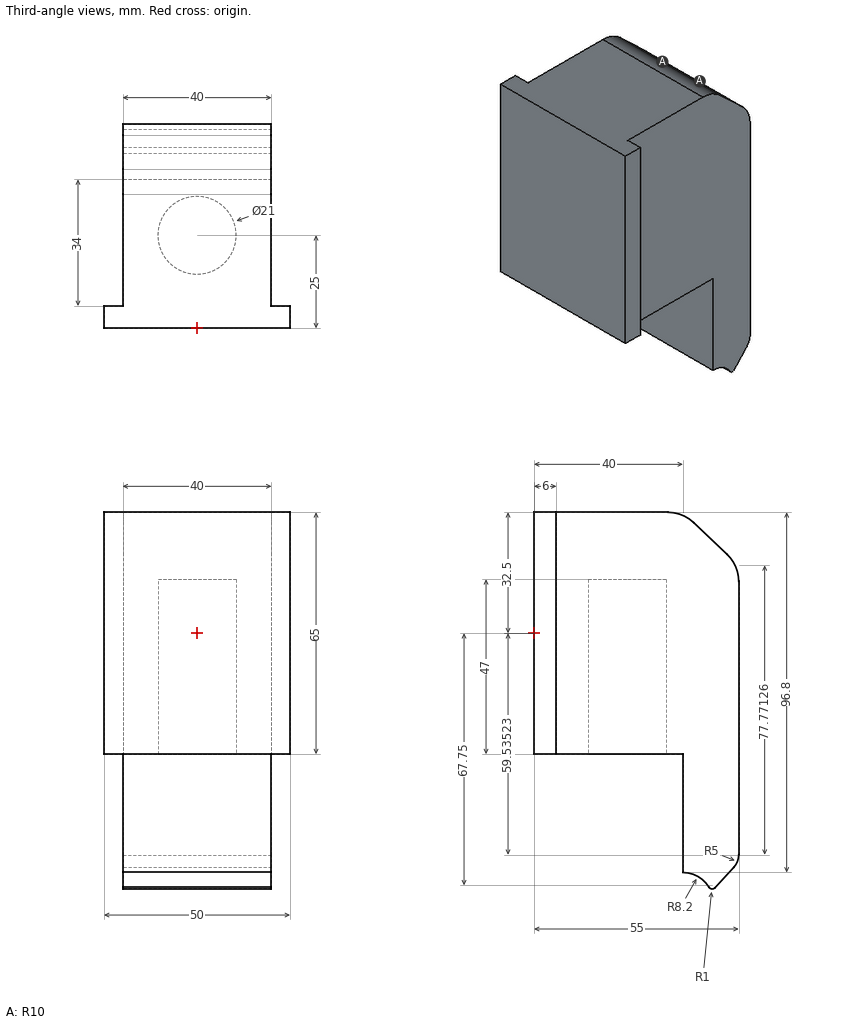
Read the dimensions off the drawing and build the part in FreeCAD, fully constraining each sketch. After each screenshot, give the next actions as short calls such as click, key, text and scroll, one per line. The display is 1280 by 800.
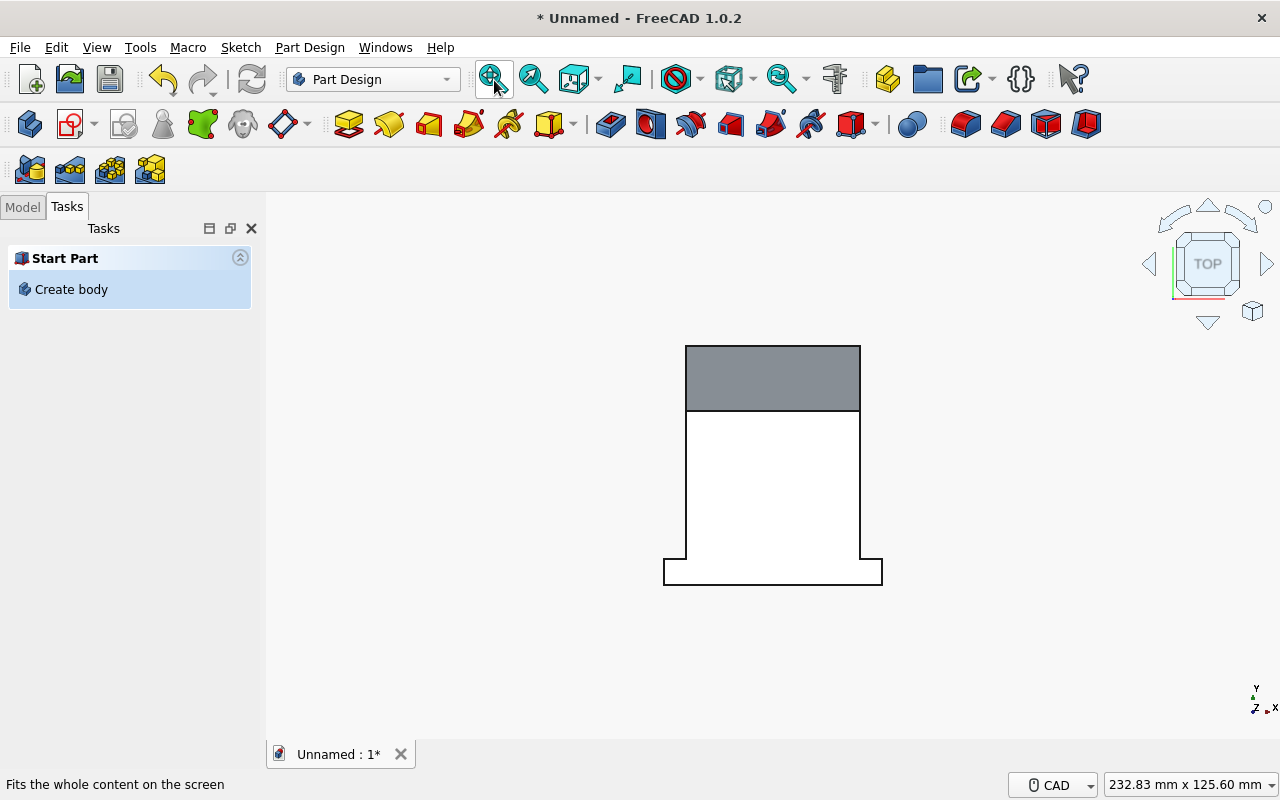
click(773, 410)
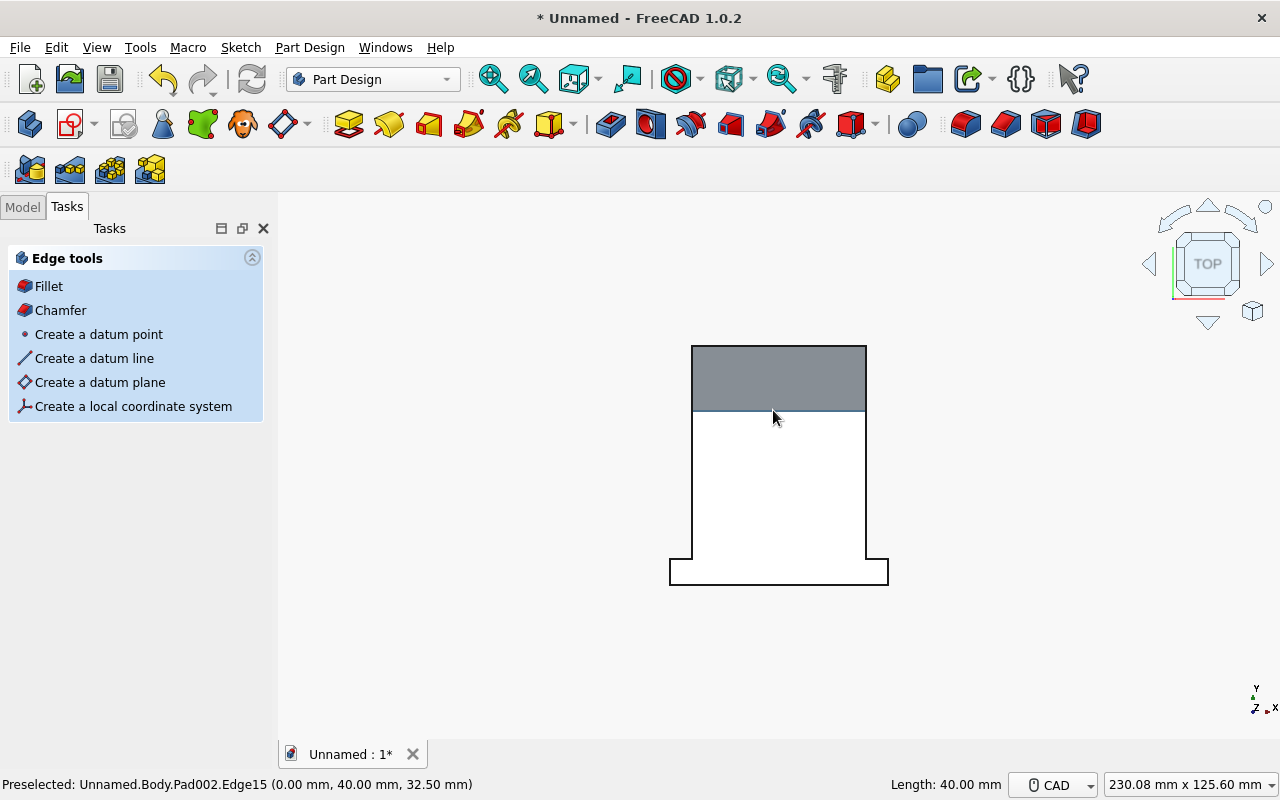
key(1)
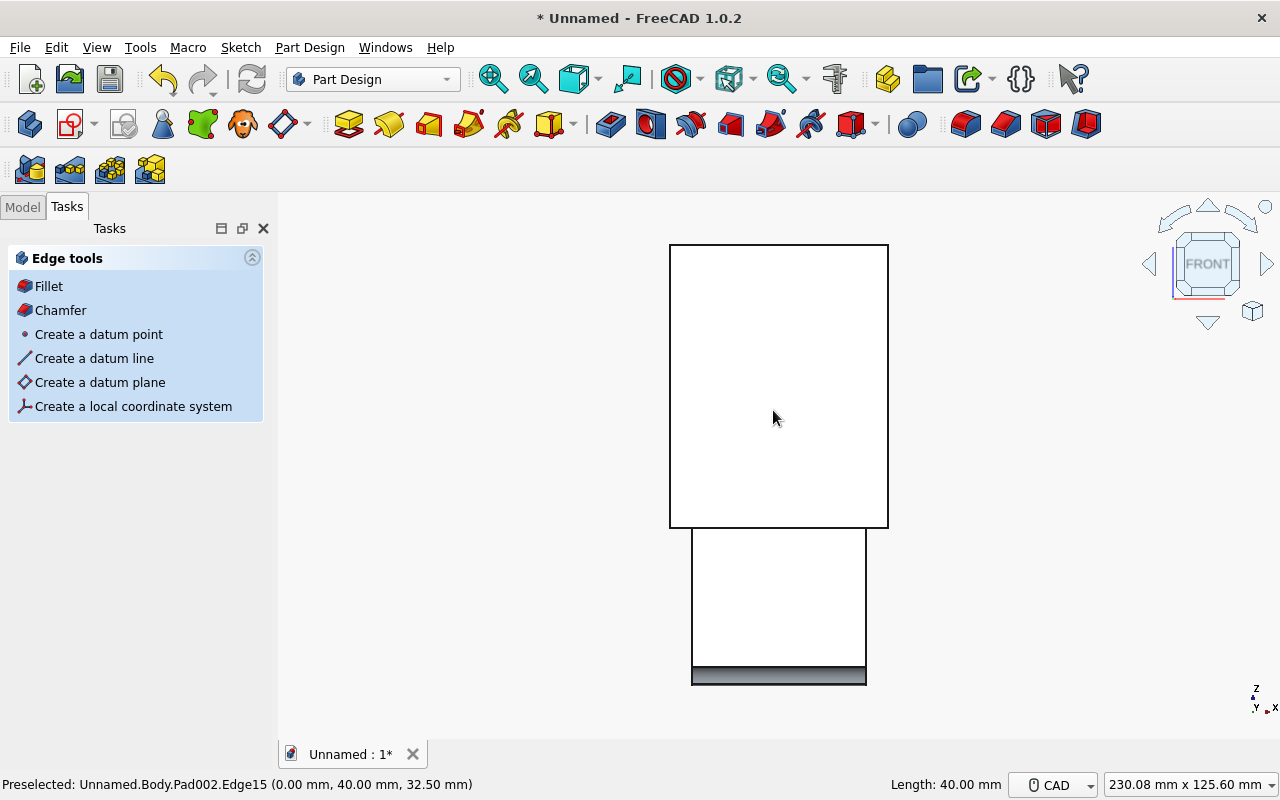
key(3)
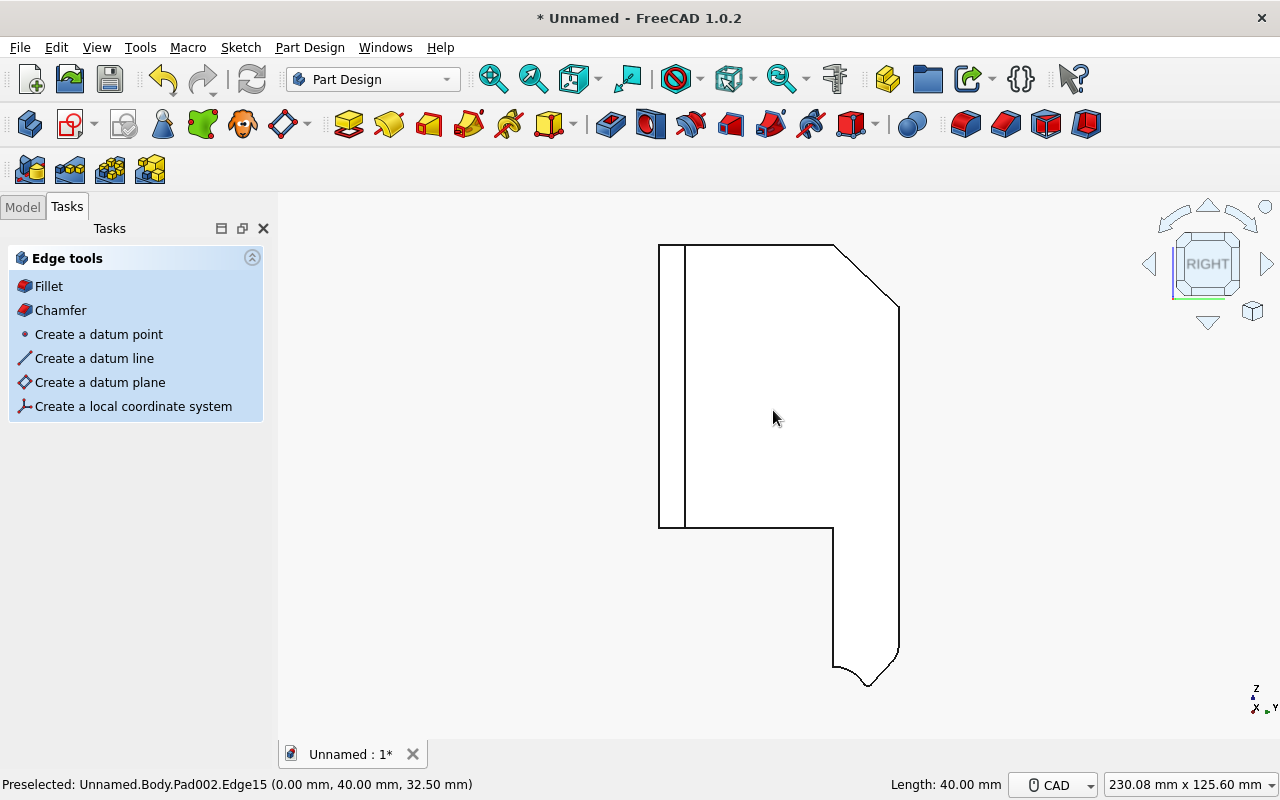
key(5)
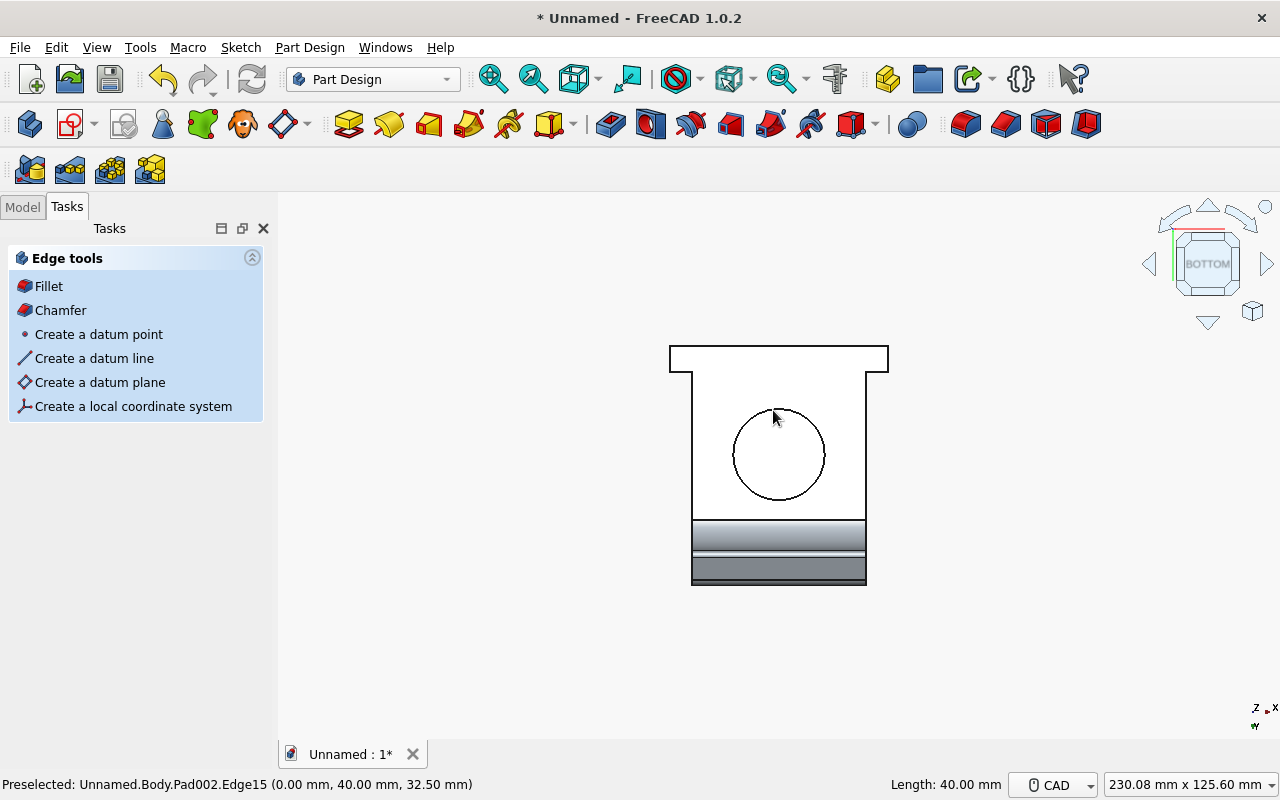
click(494, 80)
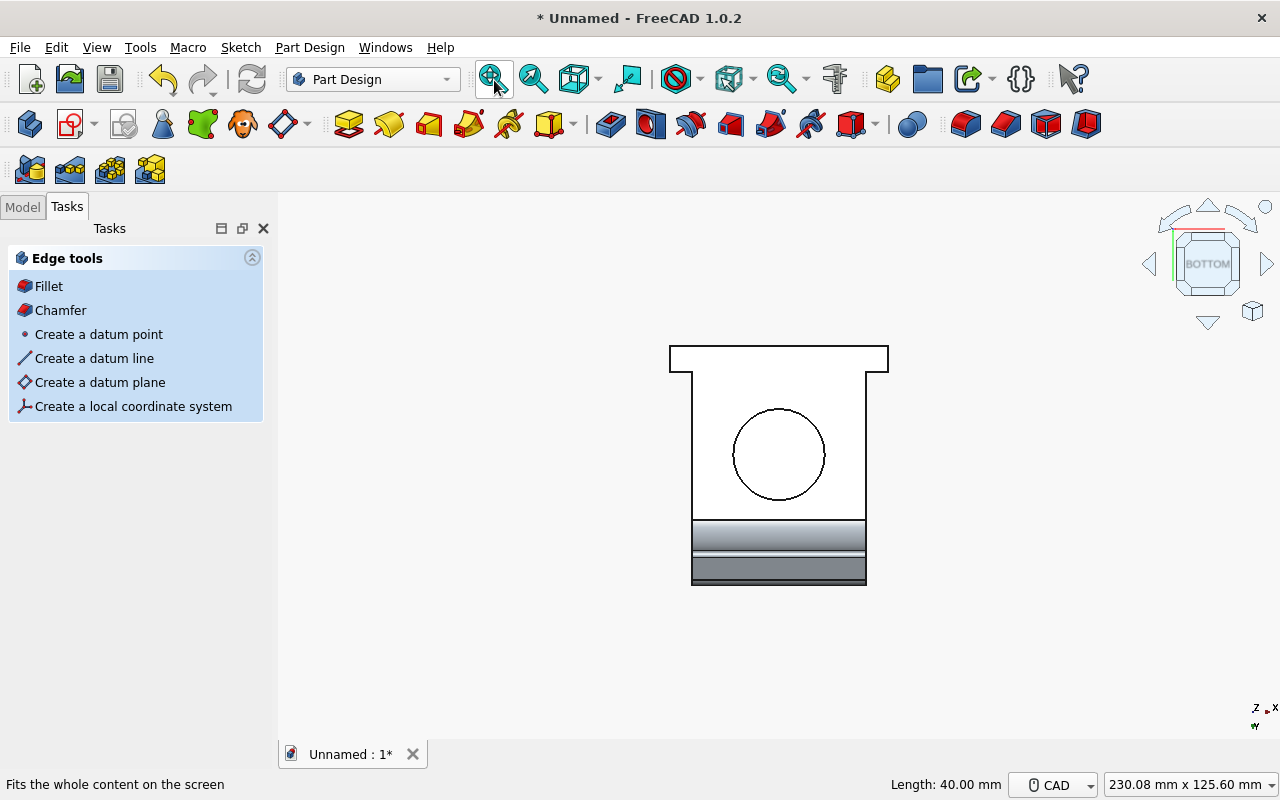
key(4)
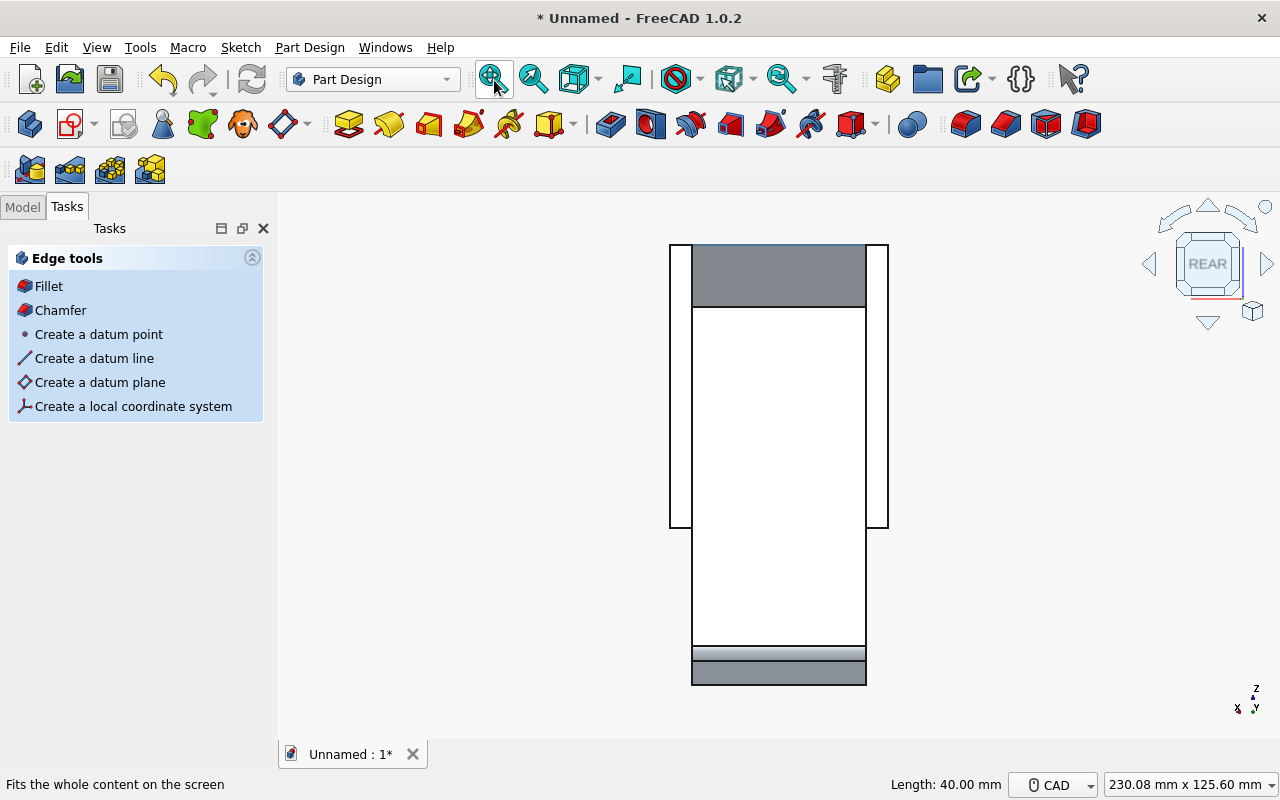
key(6)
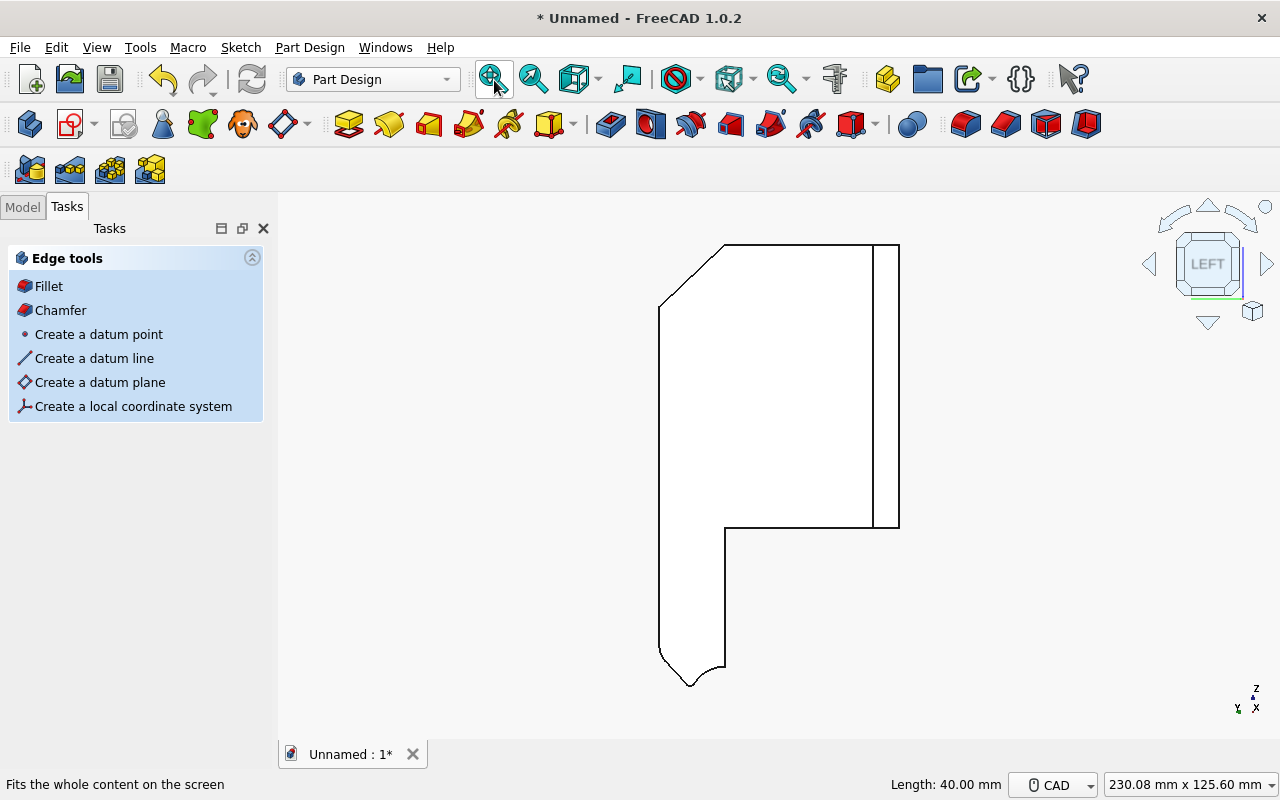
key(v)
key(3)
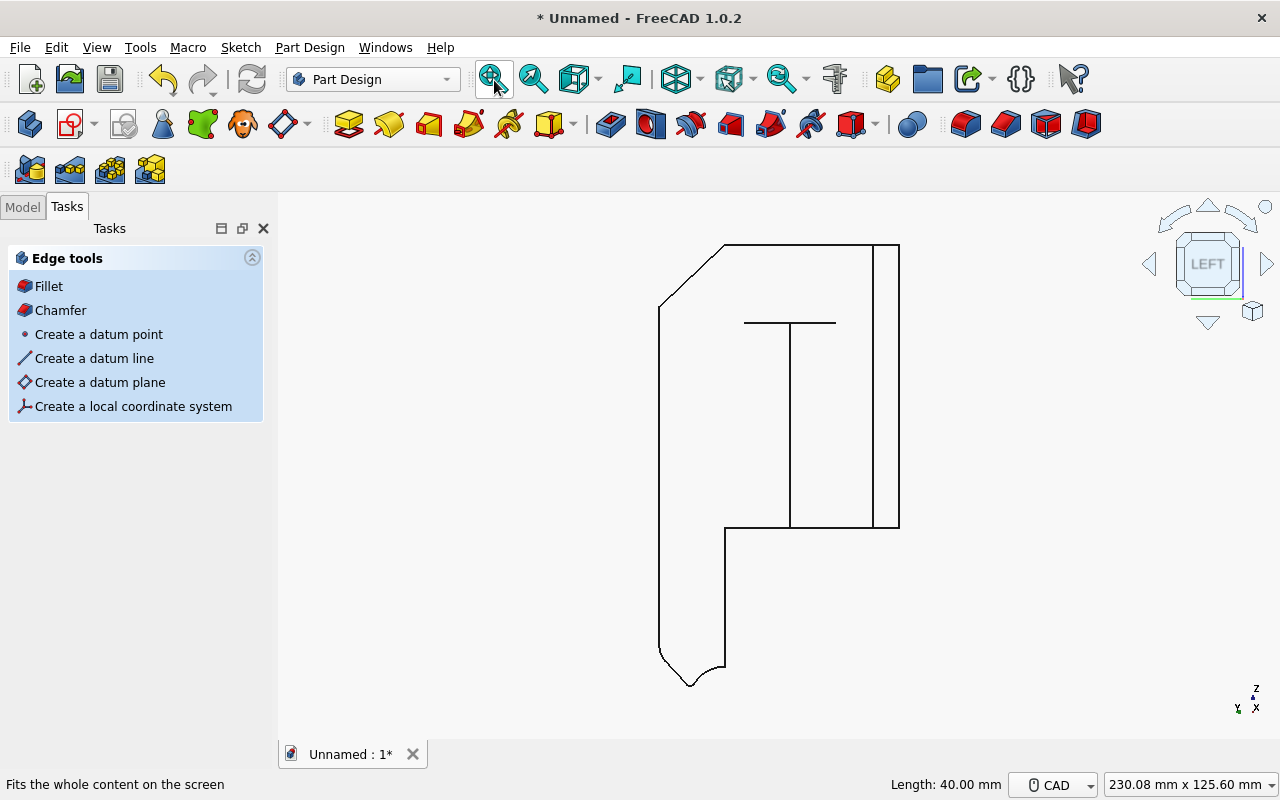
key(0)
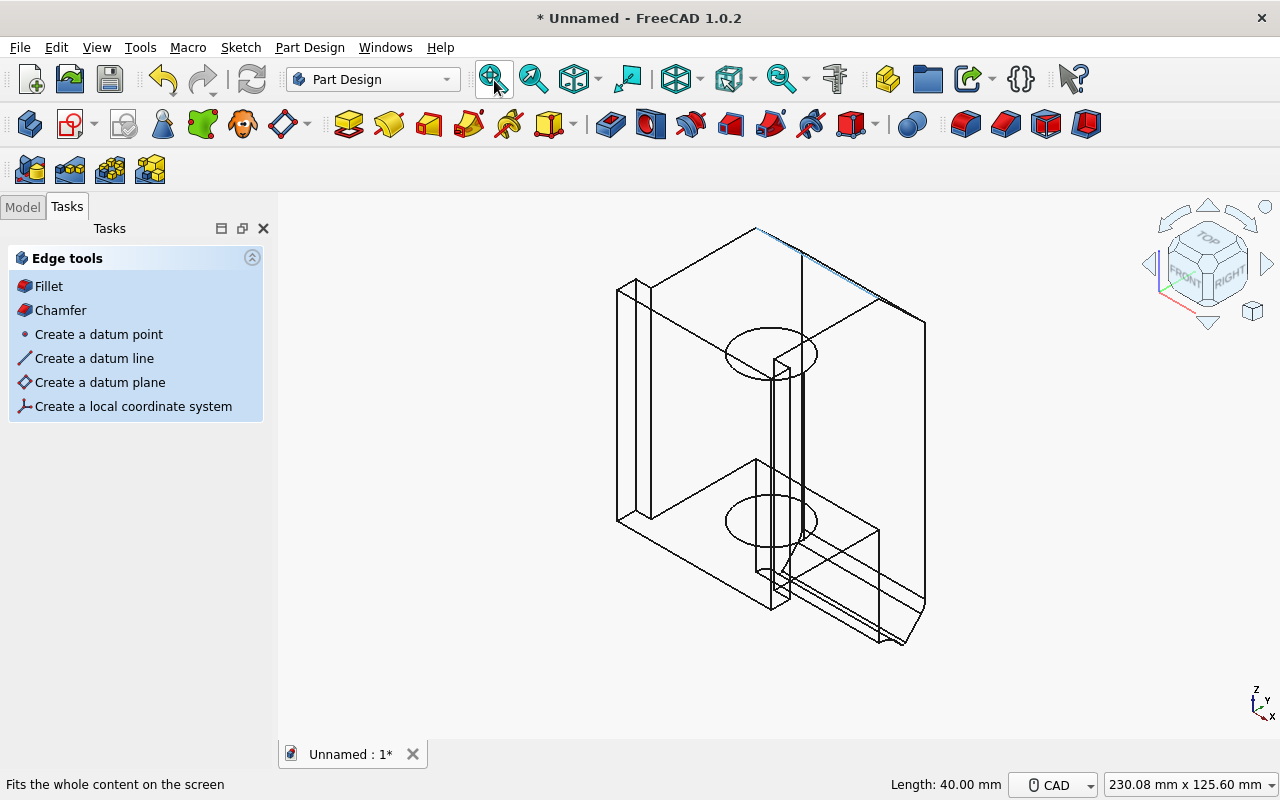
click(494, 80)